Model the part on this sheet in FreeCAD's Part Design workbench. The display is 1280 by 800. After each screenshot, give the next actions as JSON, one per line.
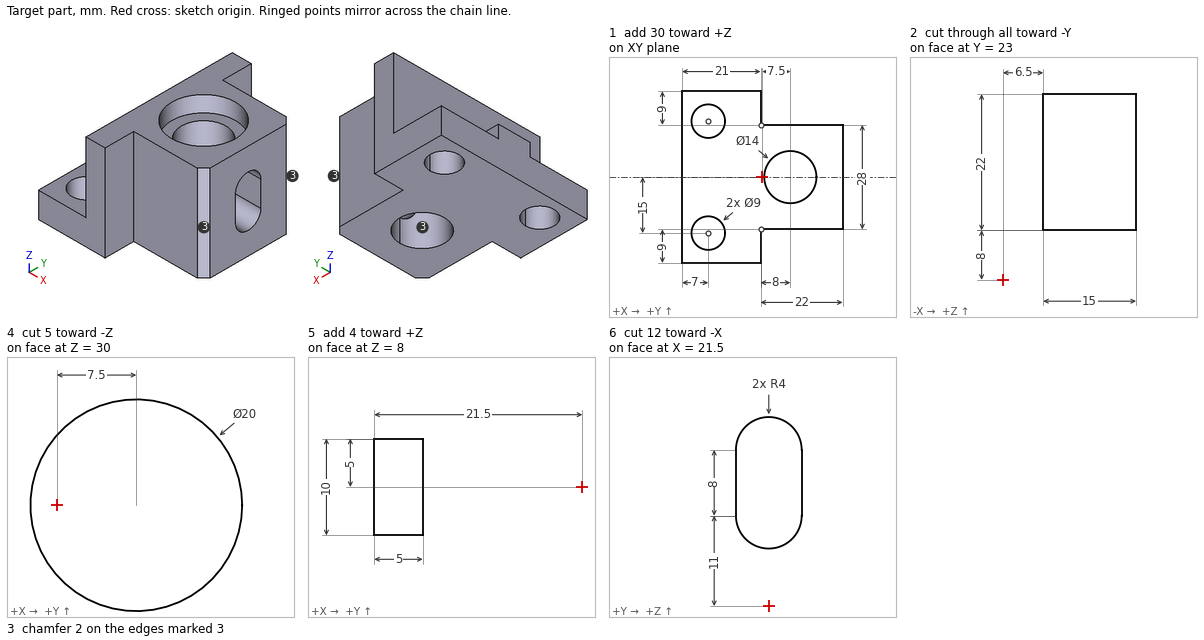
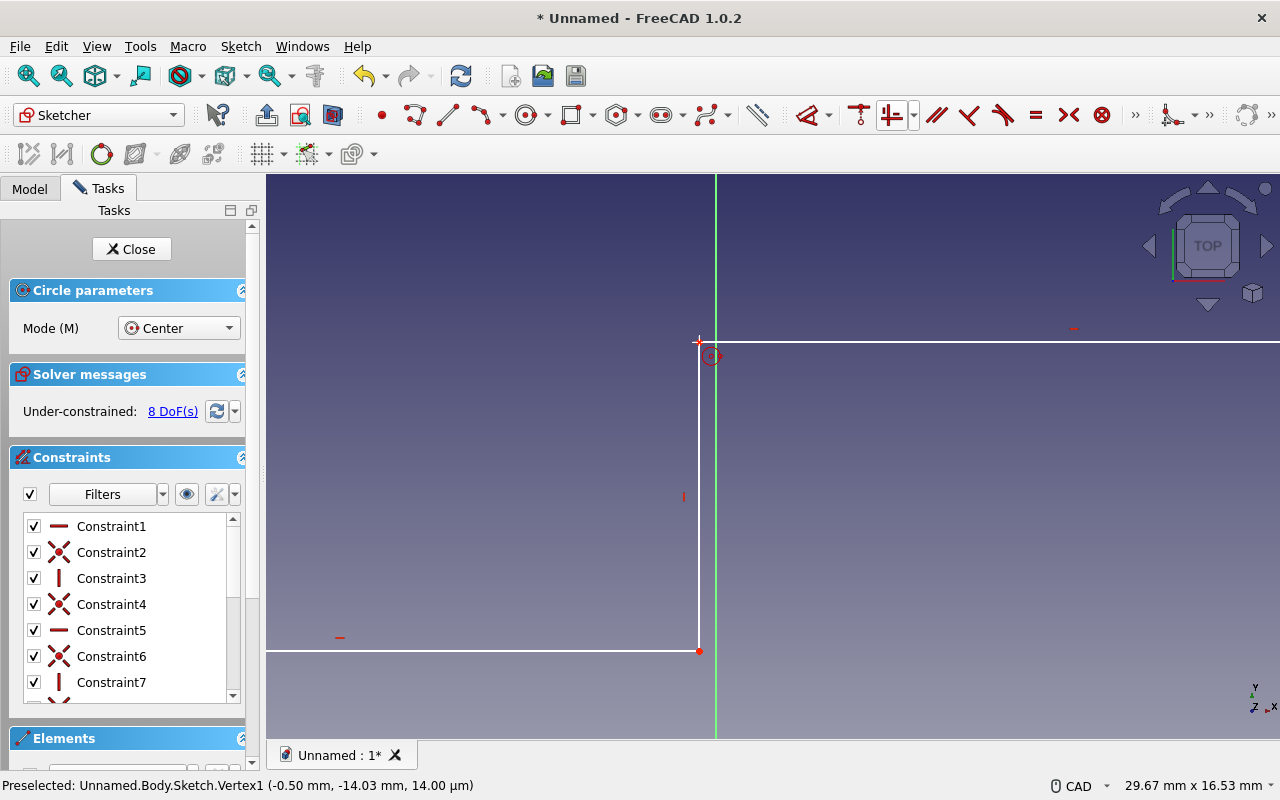
{"action": "scroll", "coordinate": [701, 651], "scroll_direction": "down", "scroll_amount": 7}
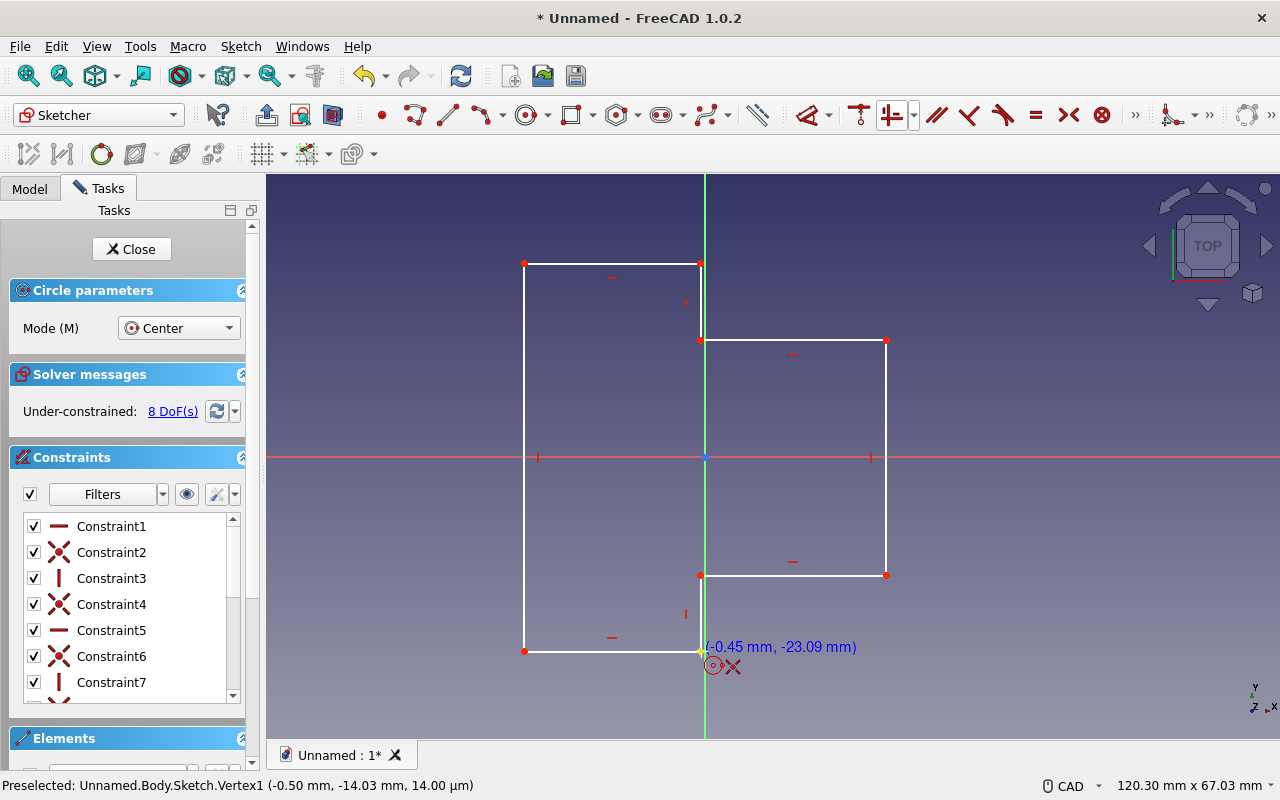
{"action": "left_click", "coordinate": [583, 584]}
{"action": "left_click", "coordinate": [610, 557]}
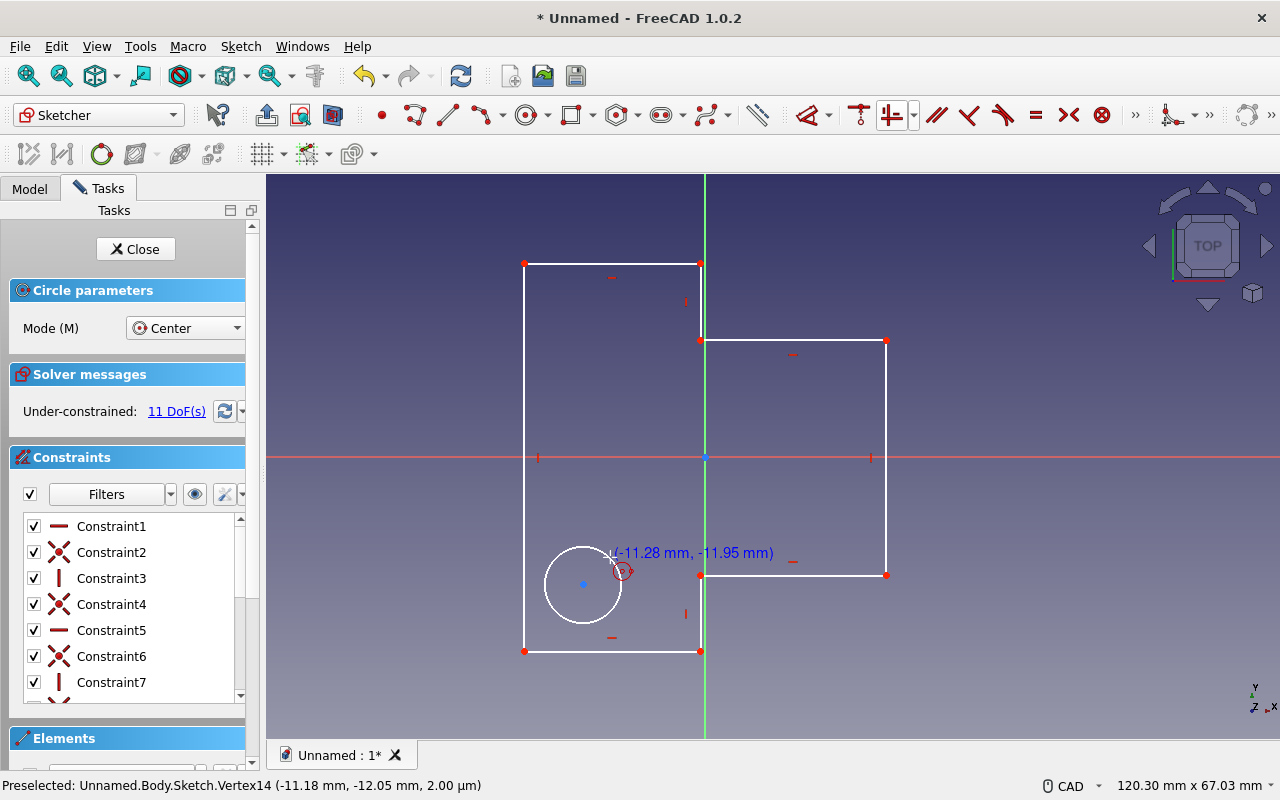
{"action": "left_click", "coordinate": [768, 457]}
{"action": "left_click", "coordinate": [810, 416]}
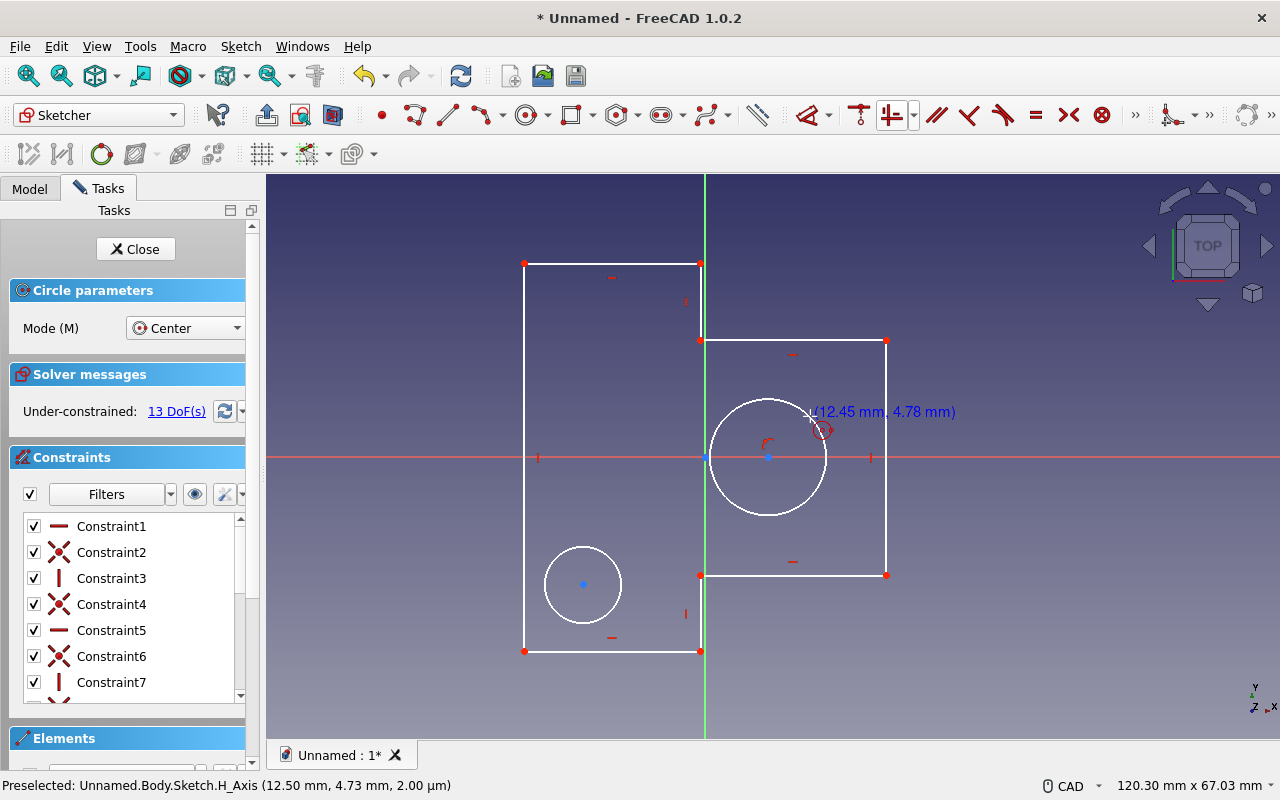
{"action": "left_click", "coordinate": [583, 331]}
{"action": "left_click", "coordinate": [610, 304]}
{"action": "key", "text": "Escape"}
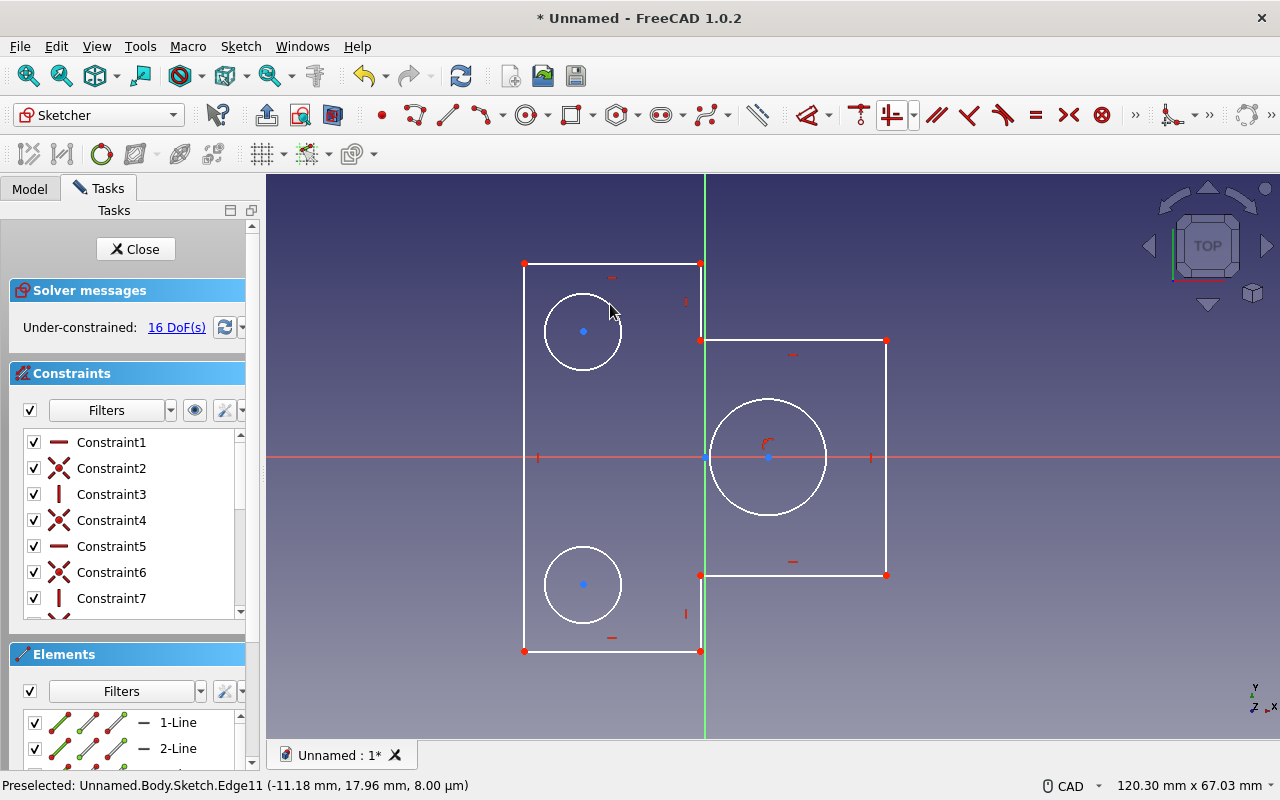
{"action": "left_click", "coordinate": [610, 558]}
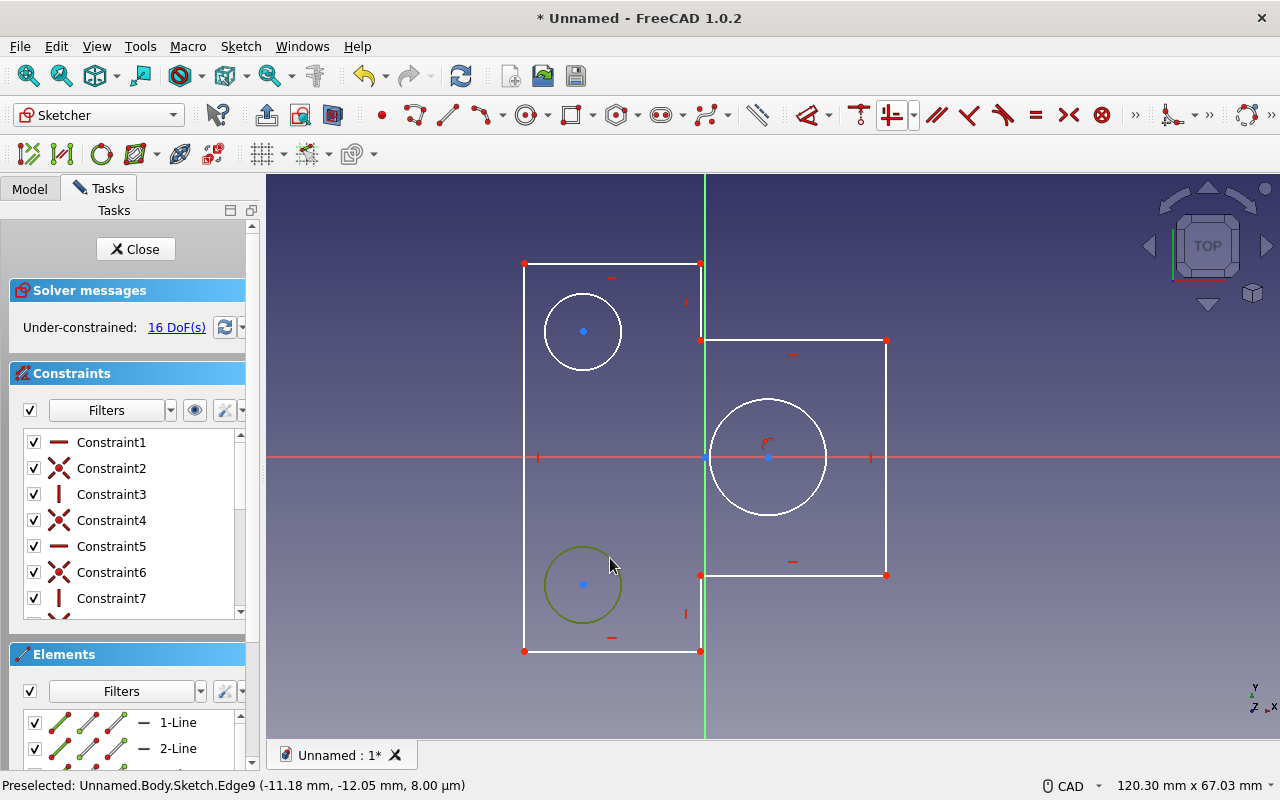
{"action": "left_click", "coordinate": [610, 305]}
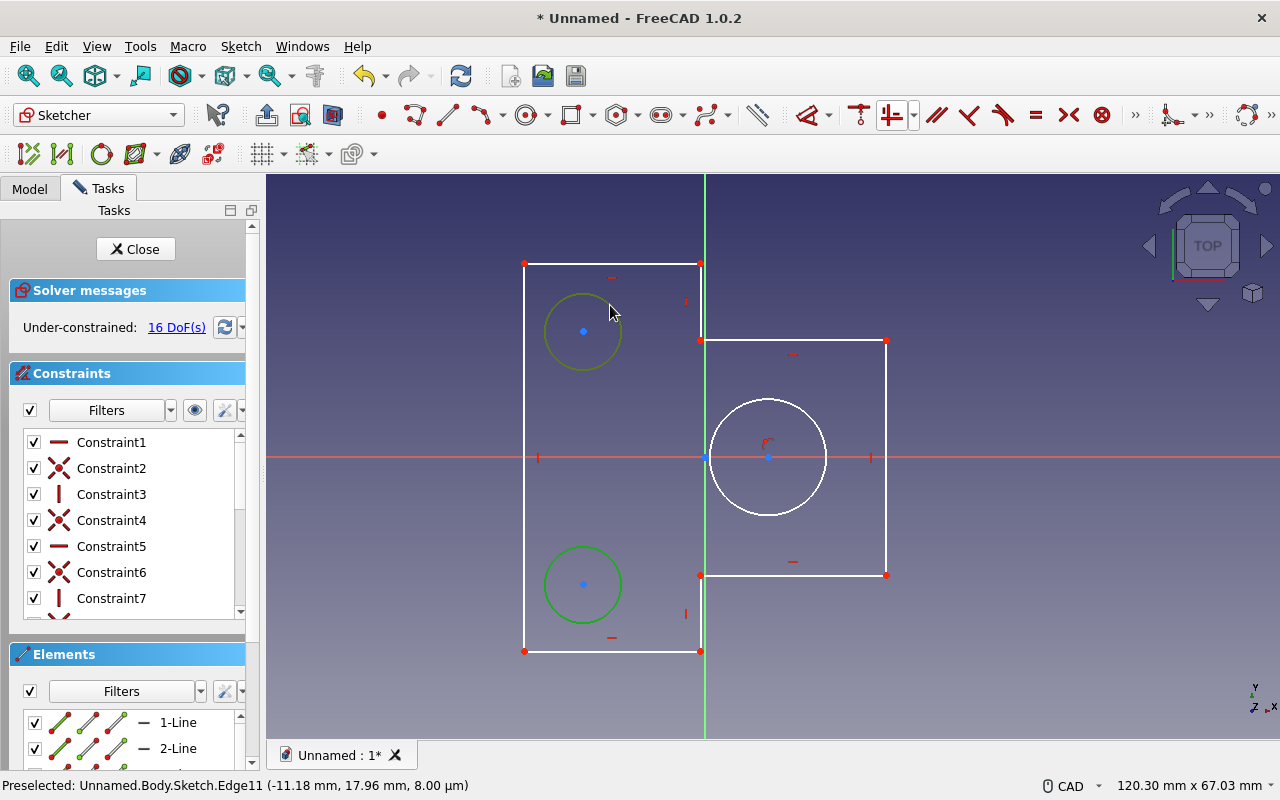
{"action": "left_click", "coordinate": [1036, 116]}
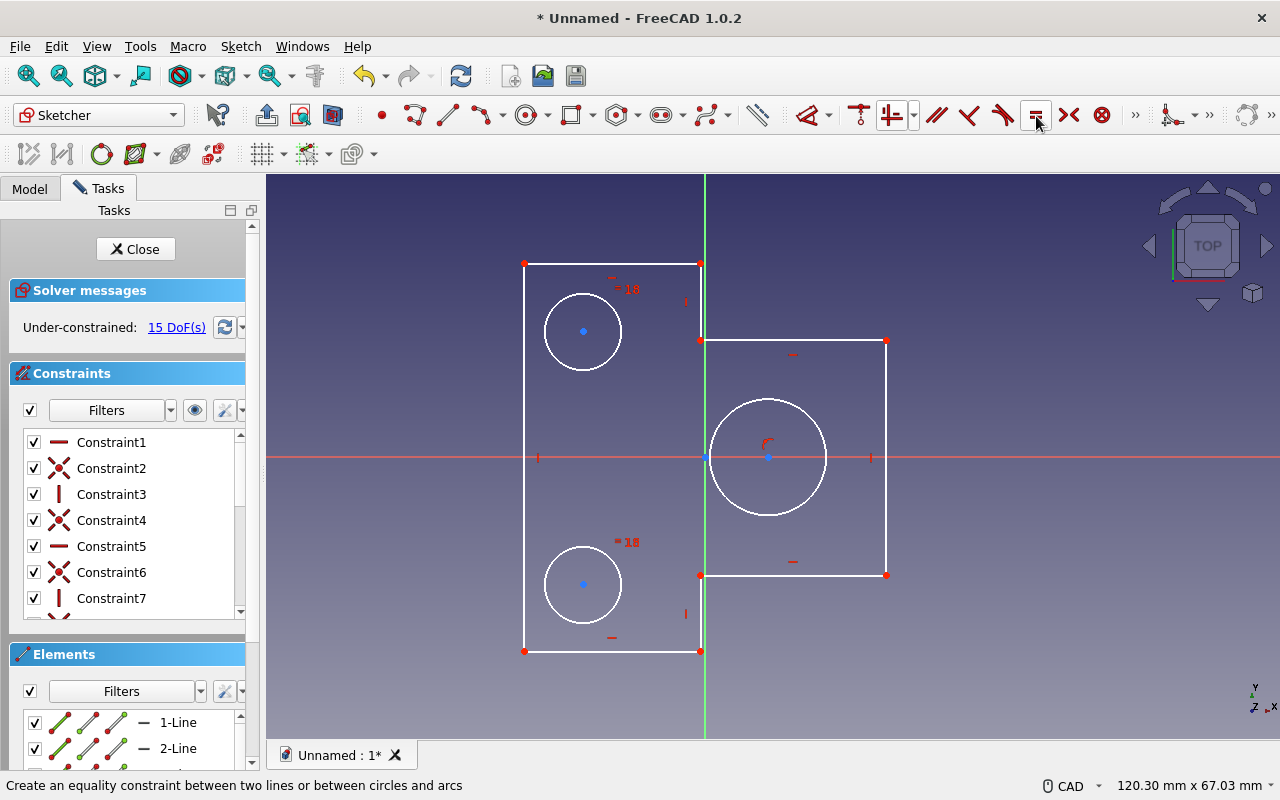
{"action": "left_click", "coordinate": [583, 585]}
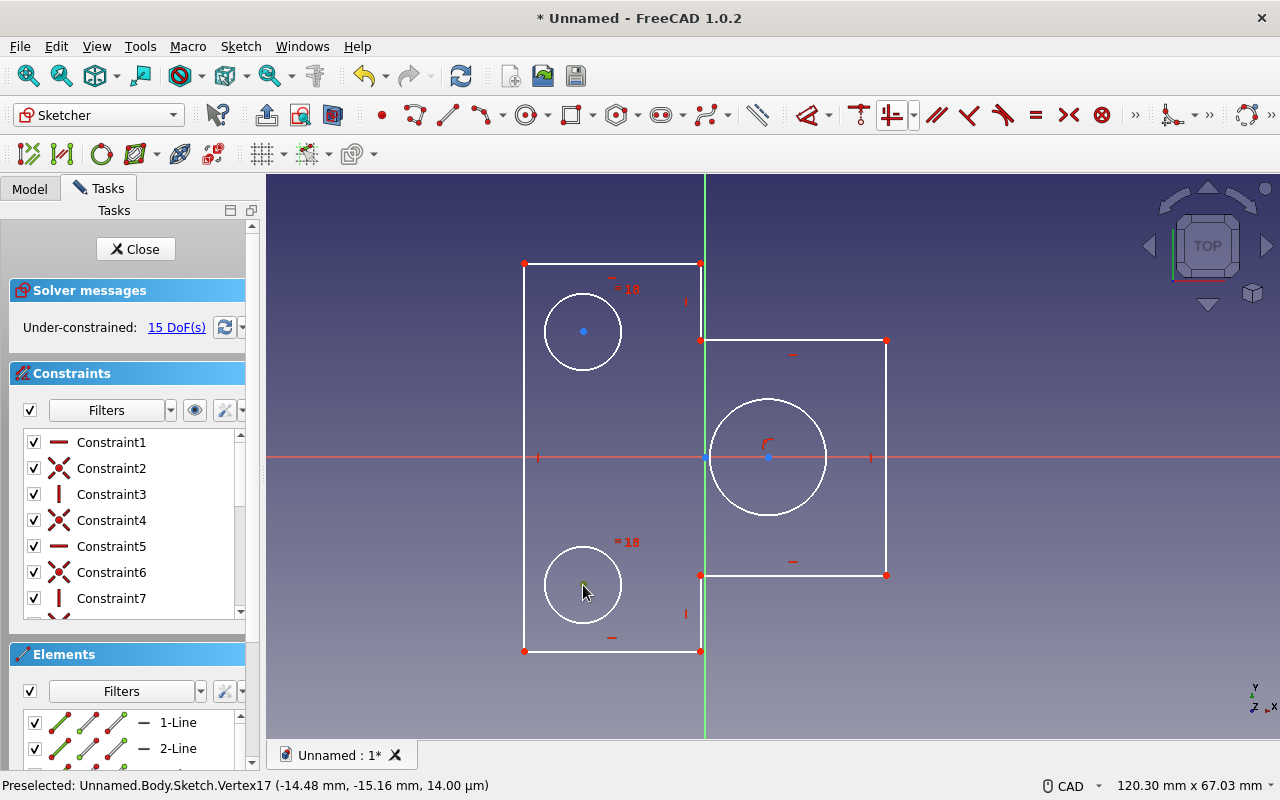
{"action": "left_click", "coordinate": [583, 332]}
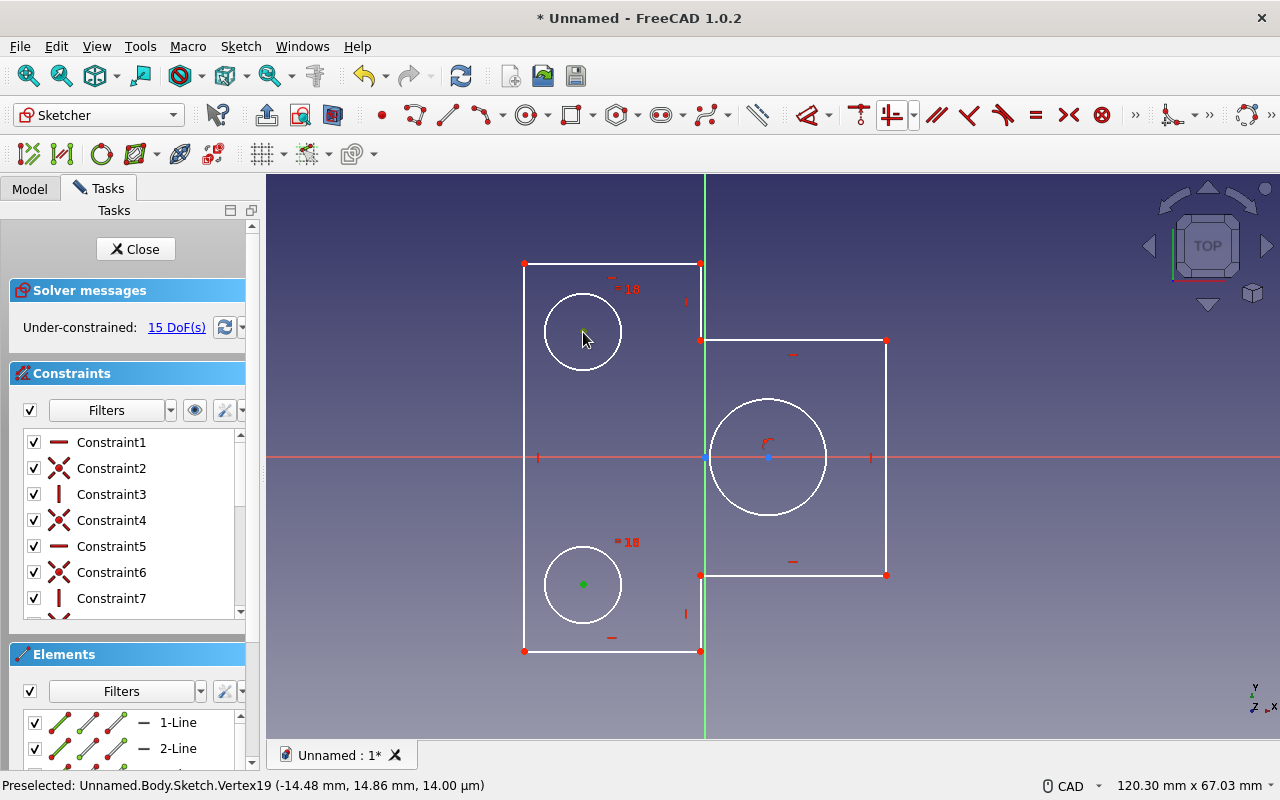
{"action": "left_click", "coordinate": [353, 457]}